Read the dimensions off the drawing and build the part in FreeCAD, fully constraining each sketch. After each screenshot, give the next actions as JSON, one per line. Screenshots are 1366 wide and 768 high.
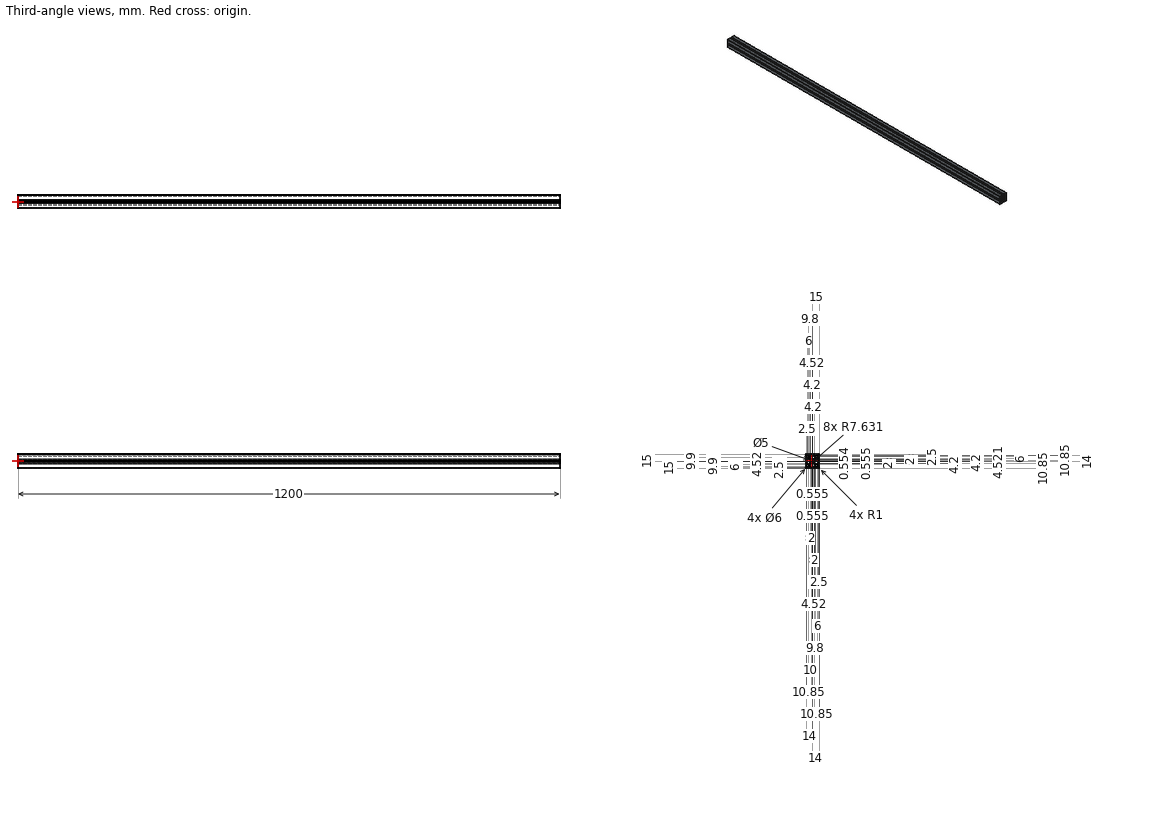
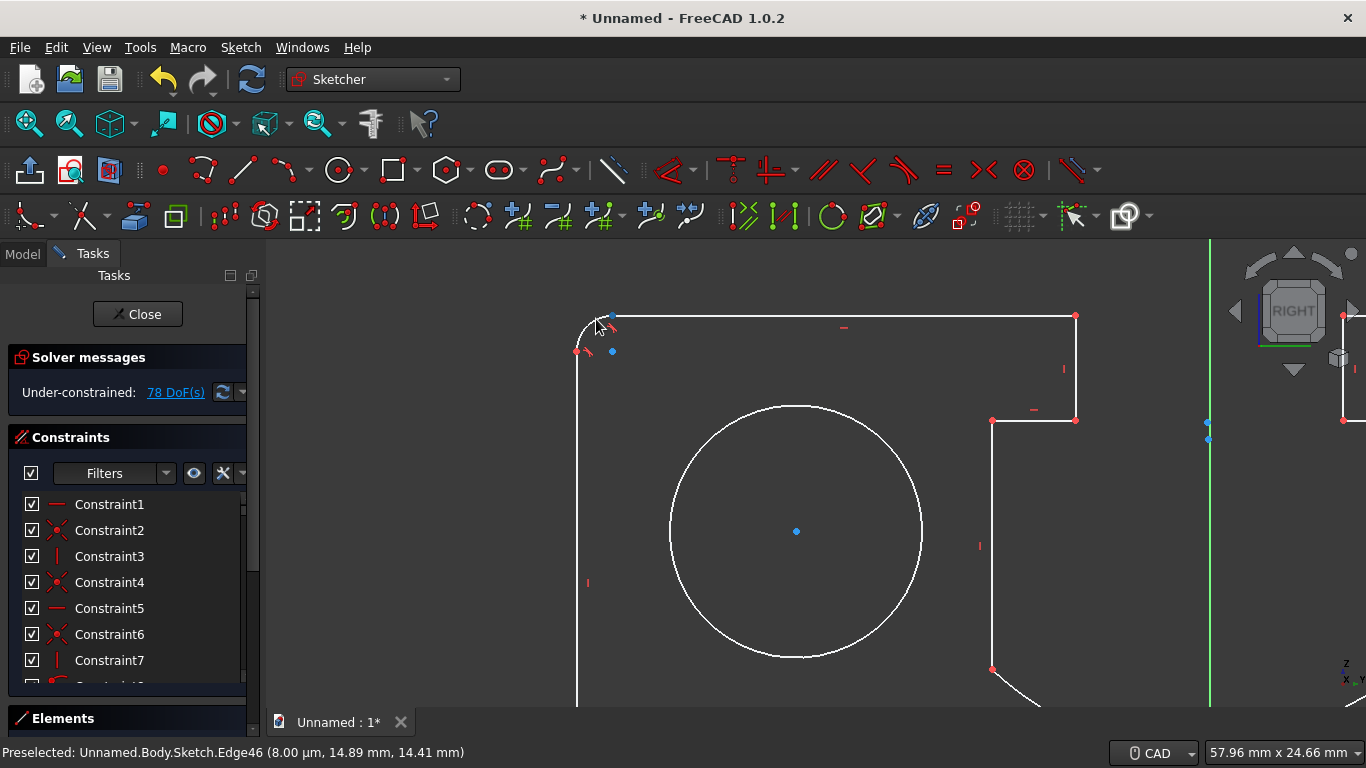
{"action": "left_click", "coordinate": [596, 320]}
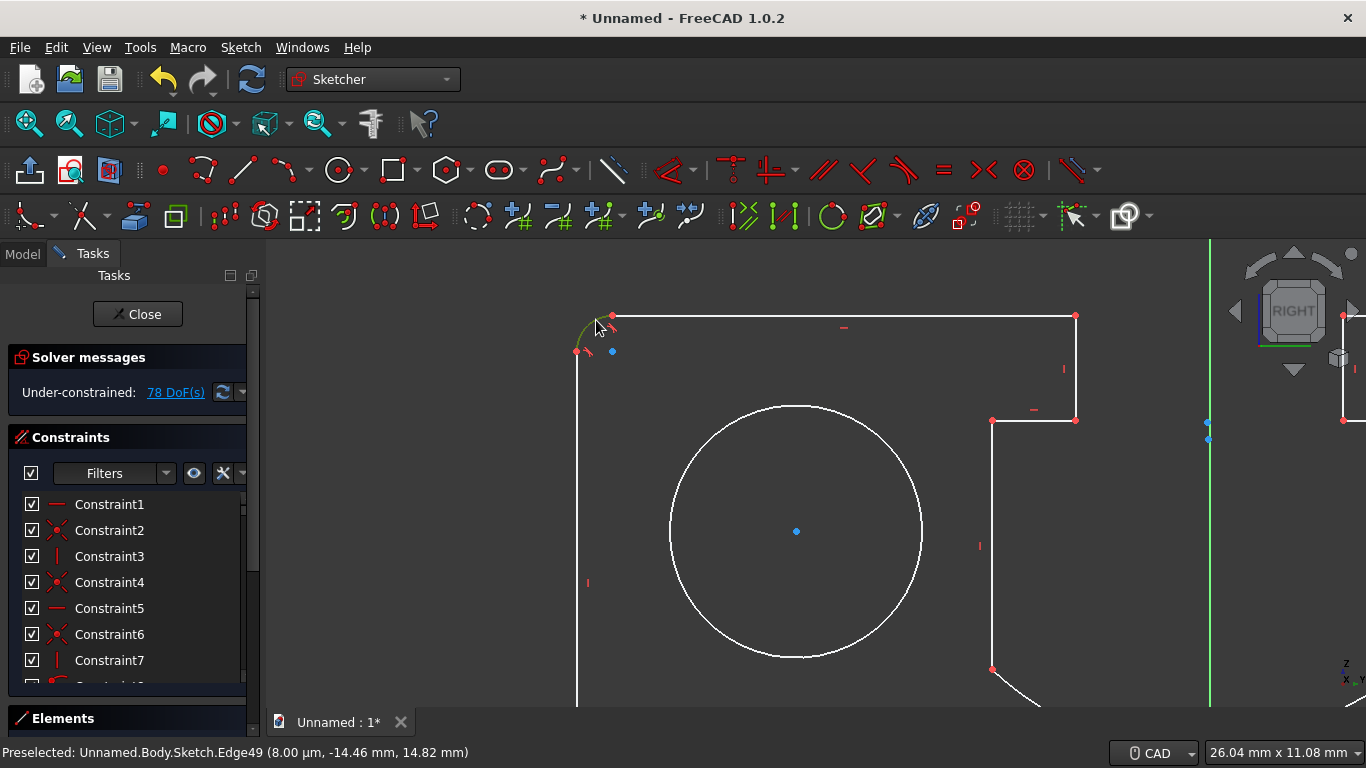
{"action": "scroll", "coordinate": [596, 319], "scroll_direction": "down", "scroll_amount": 7}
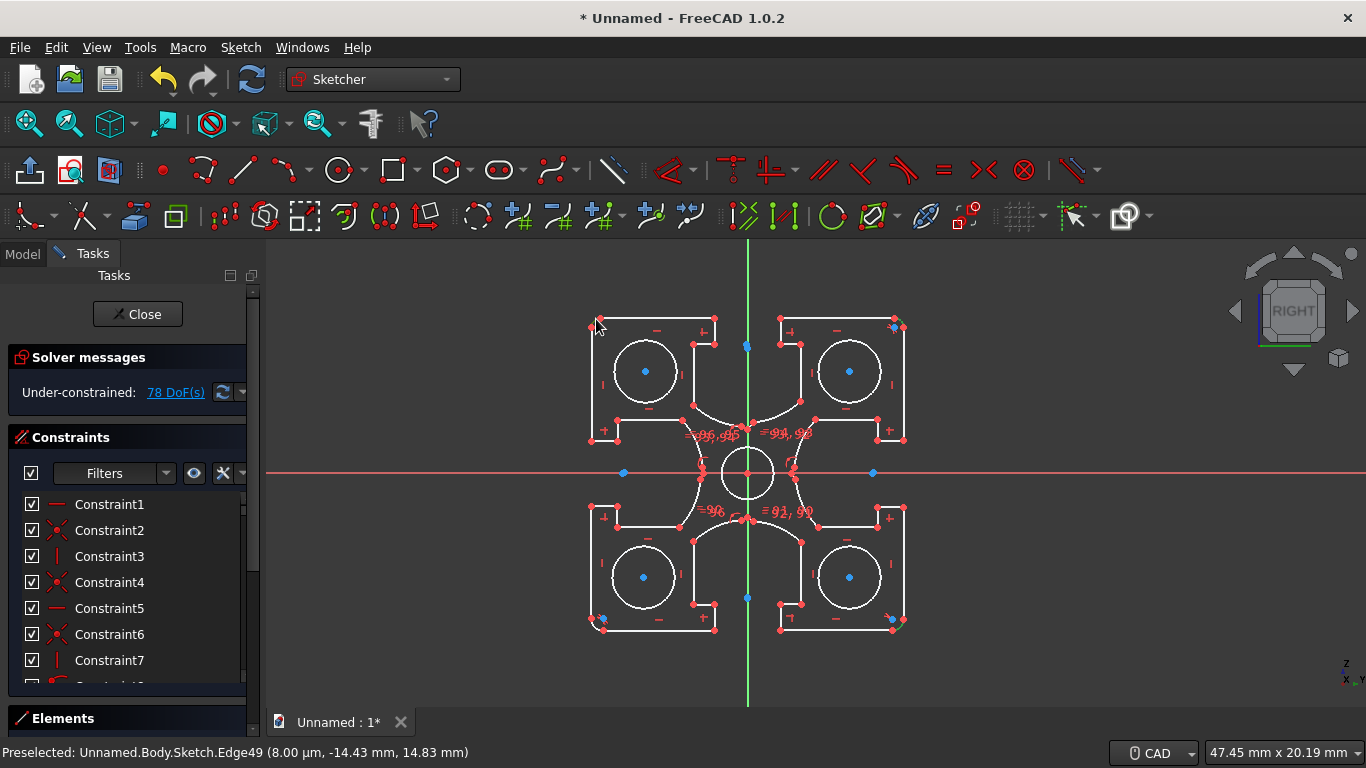
{"action": "scroll", "coordinate": [592, 624], "scroll_direction": "up", "scroll_amount": 5}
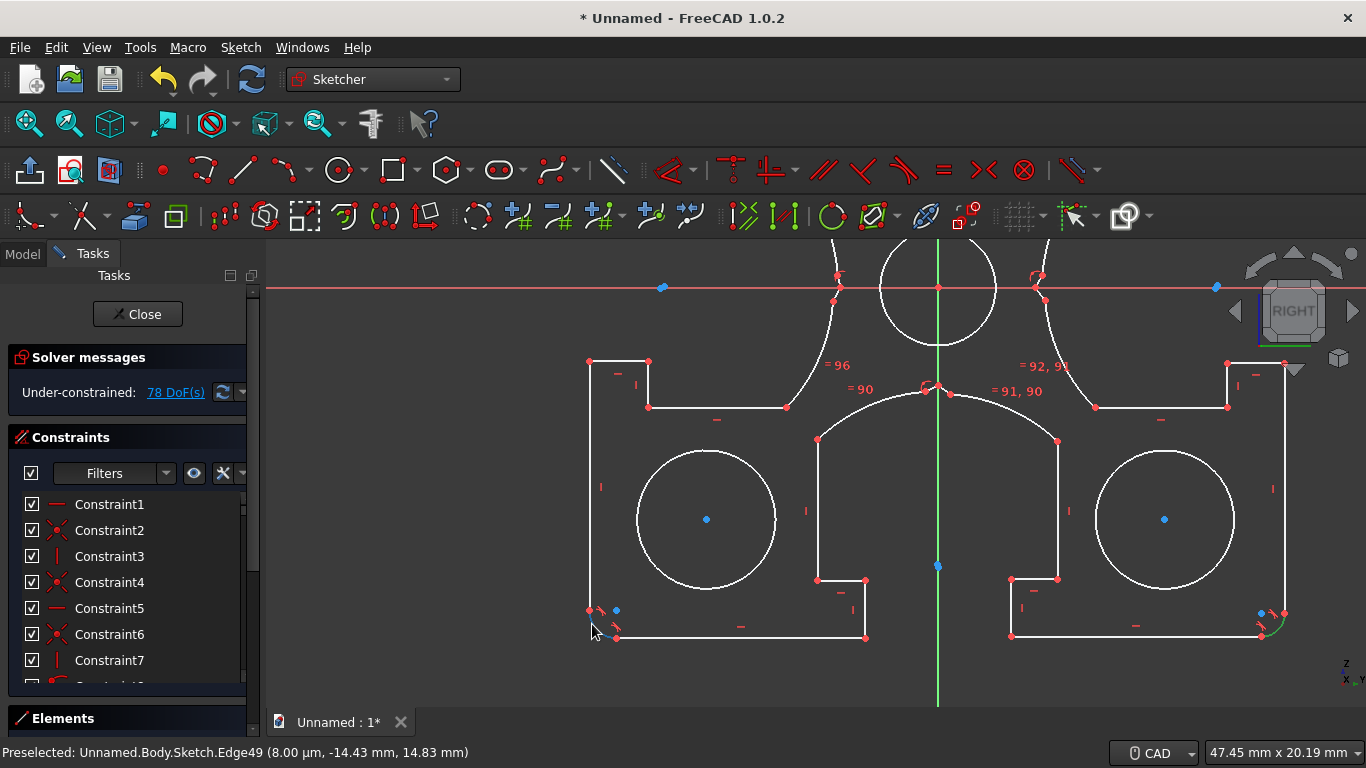
{"action": "left_click", "coordinate": [593, 623]}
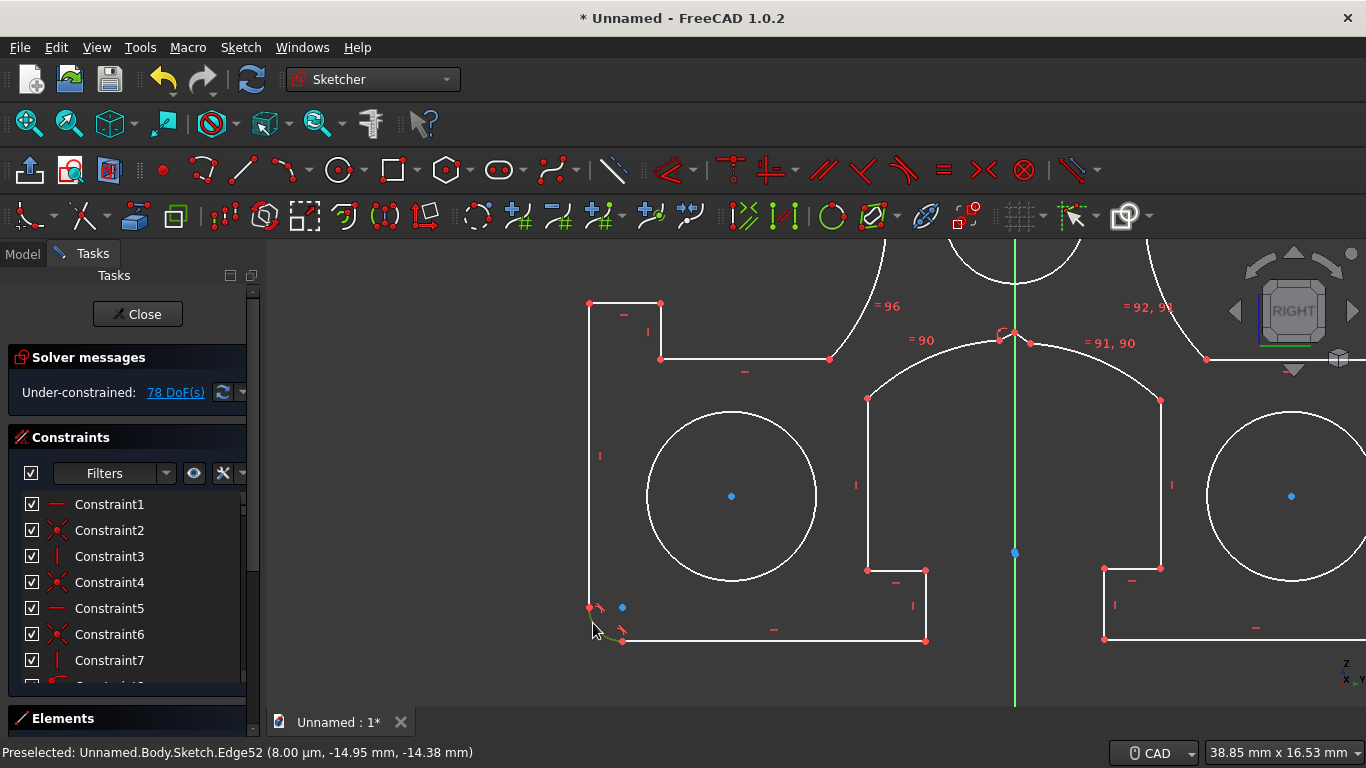
{"action": "left_click", "coordinate": [944, 170]}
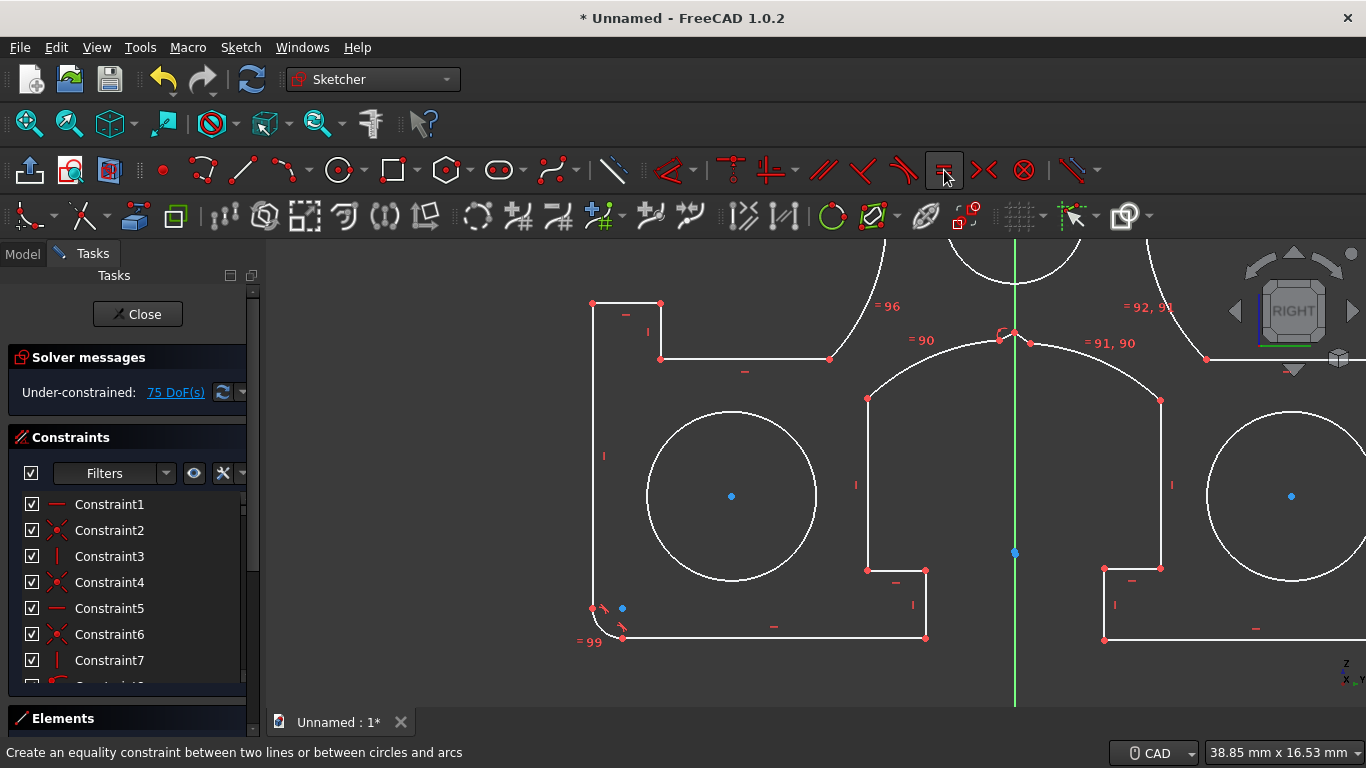
{"action": "left_click", "coordinate": [791, 436]}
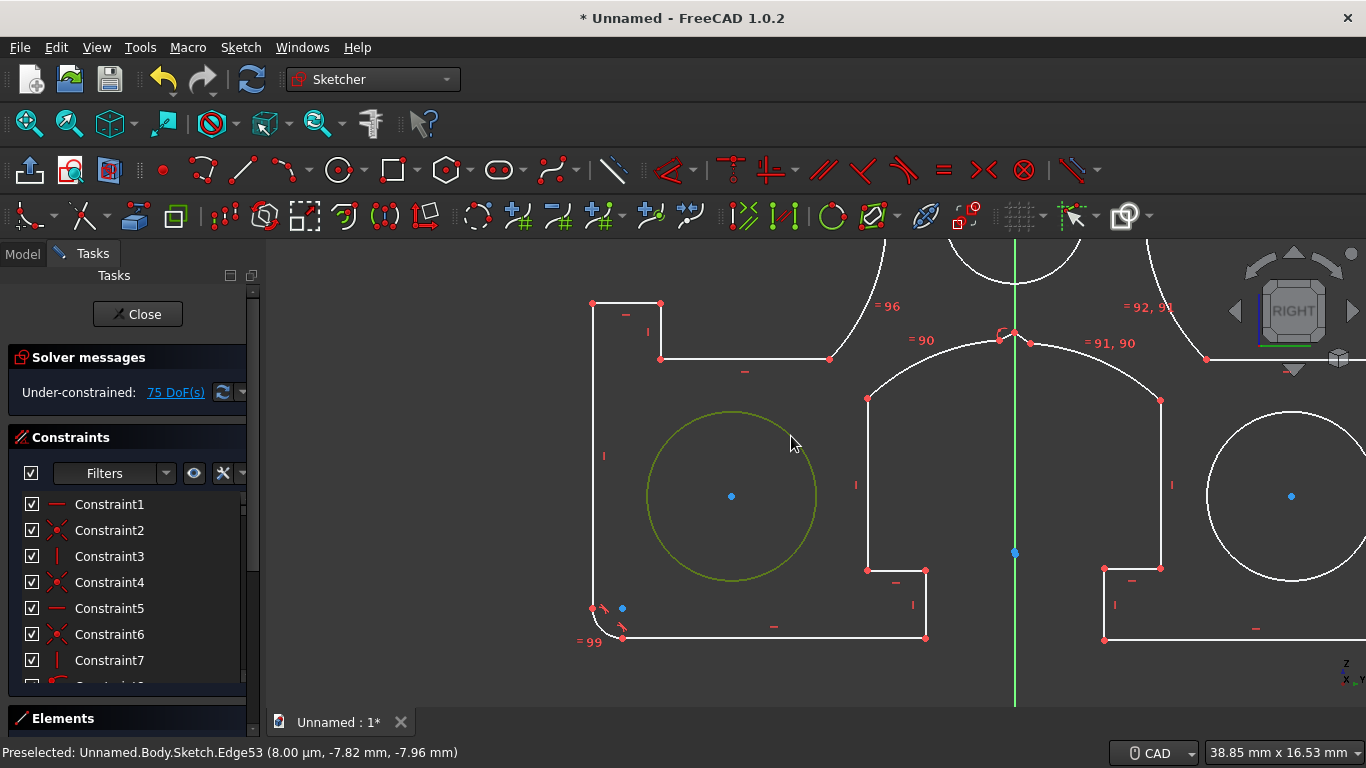
{"action": "scroll", "coordinate": [592, 624], "scroll_direction": "down", "scroll_amount": 5}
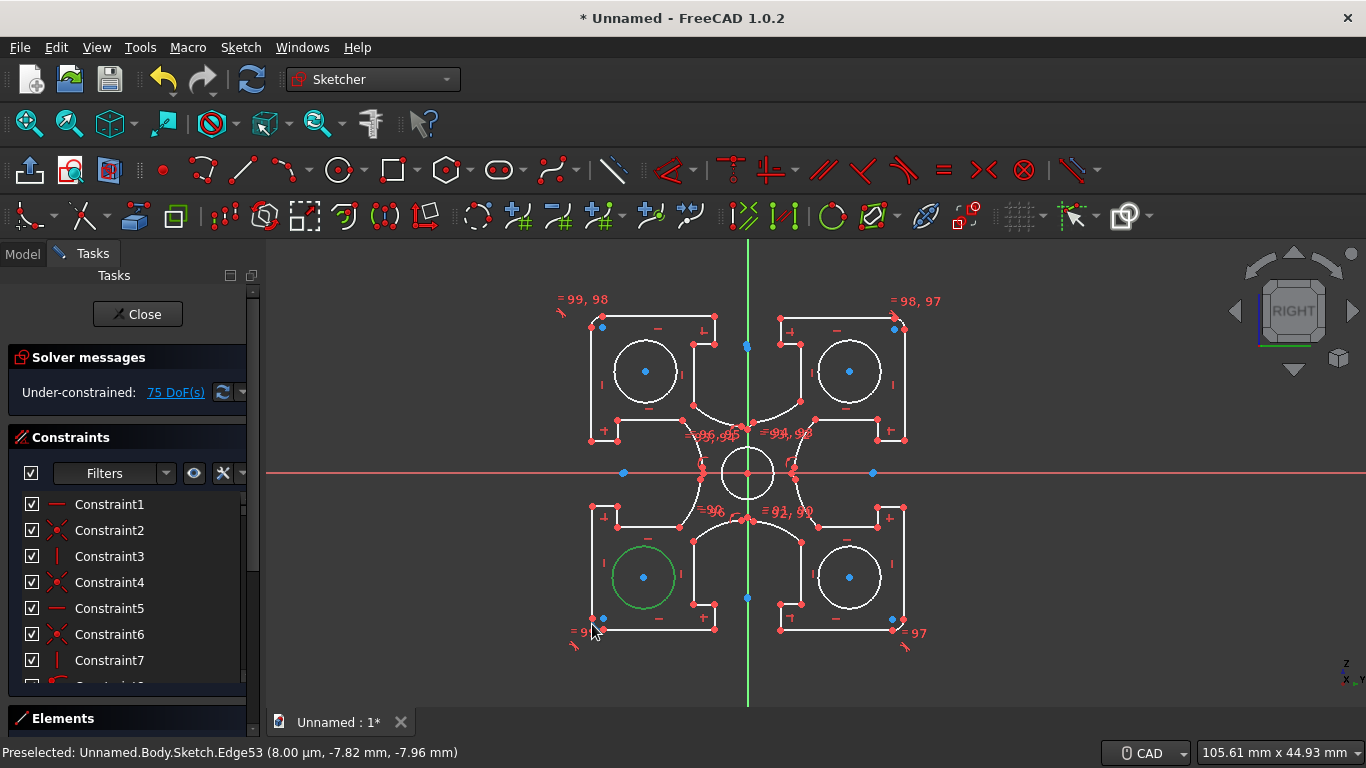
{"action": "left_click", "coordinate": [871, 555]}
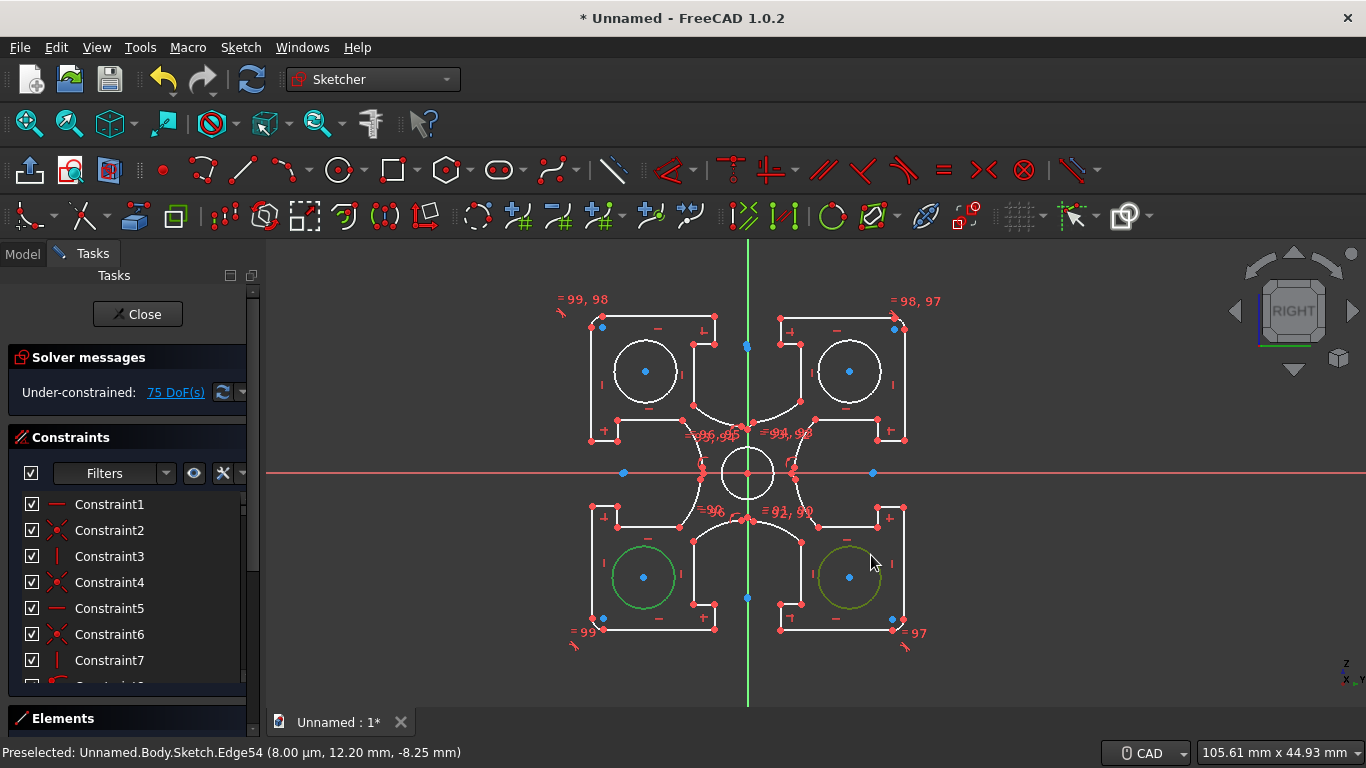
{"action": "left_click", "coordinate": [667, 349]}